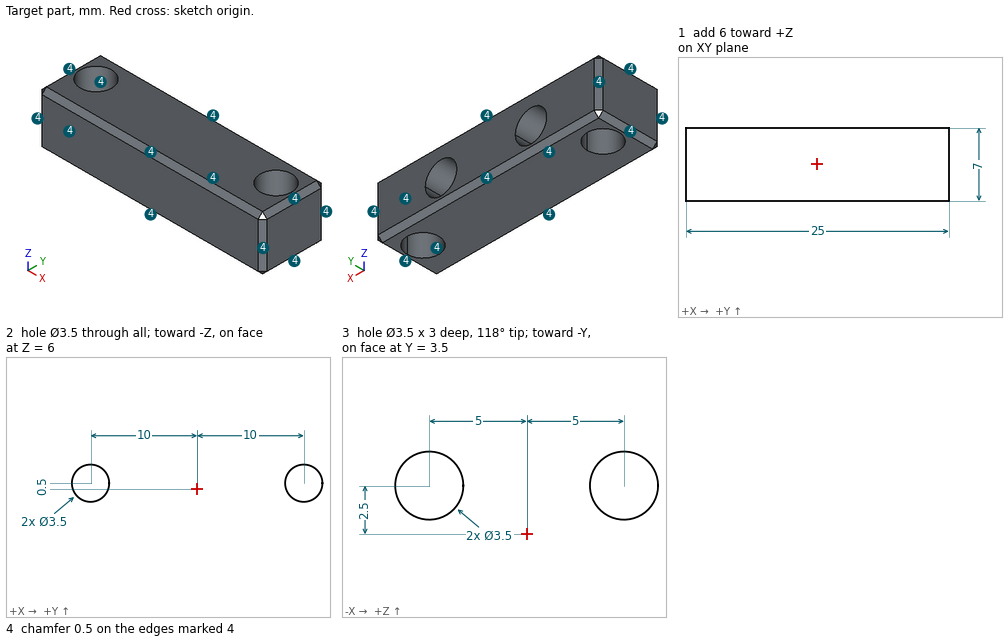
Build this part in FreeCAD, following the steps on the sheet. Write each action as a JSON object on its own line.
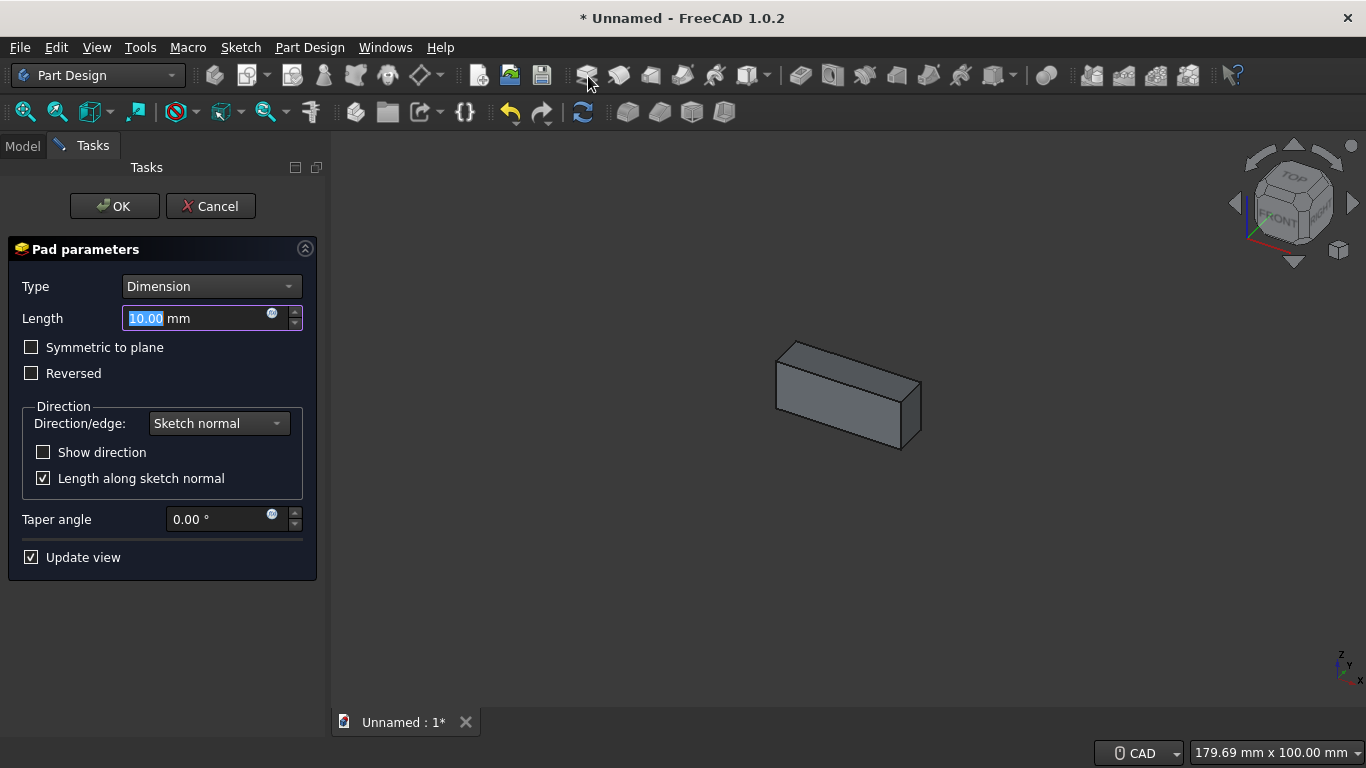
{"action": "type", "text": "6"}
{"action": "key", "text": "Tab"}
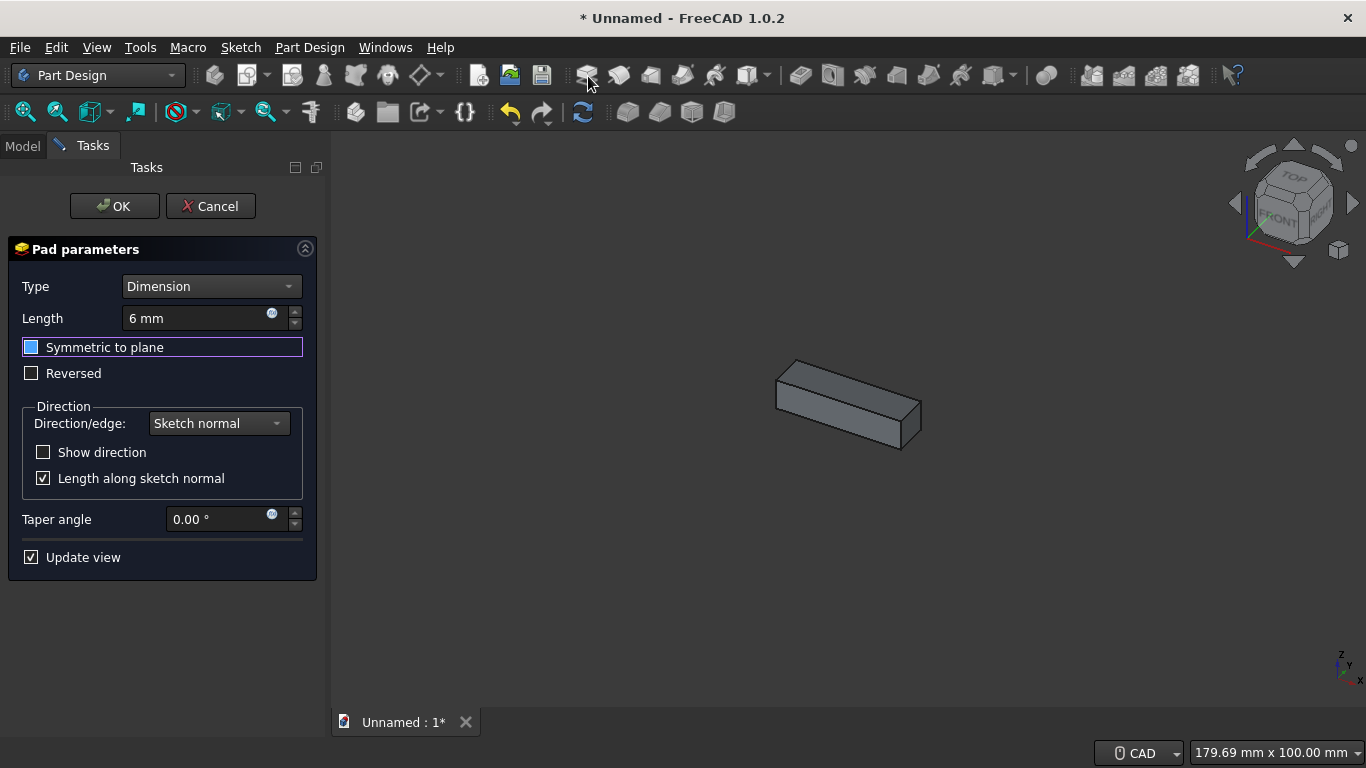
{"action": "left_click", "coordinate": [115, 206]}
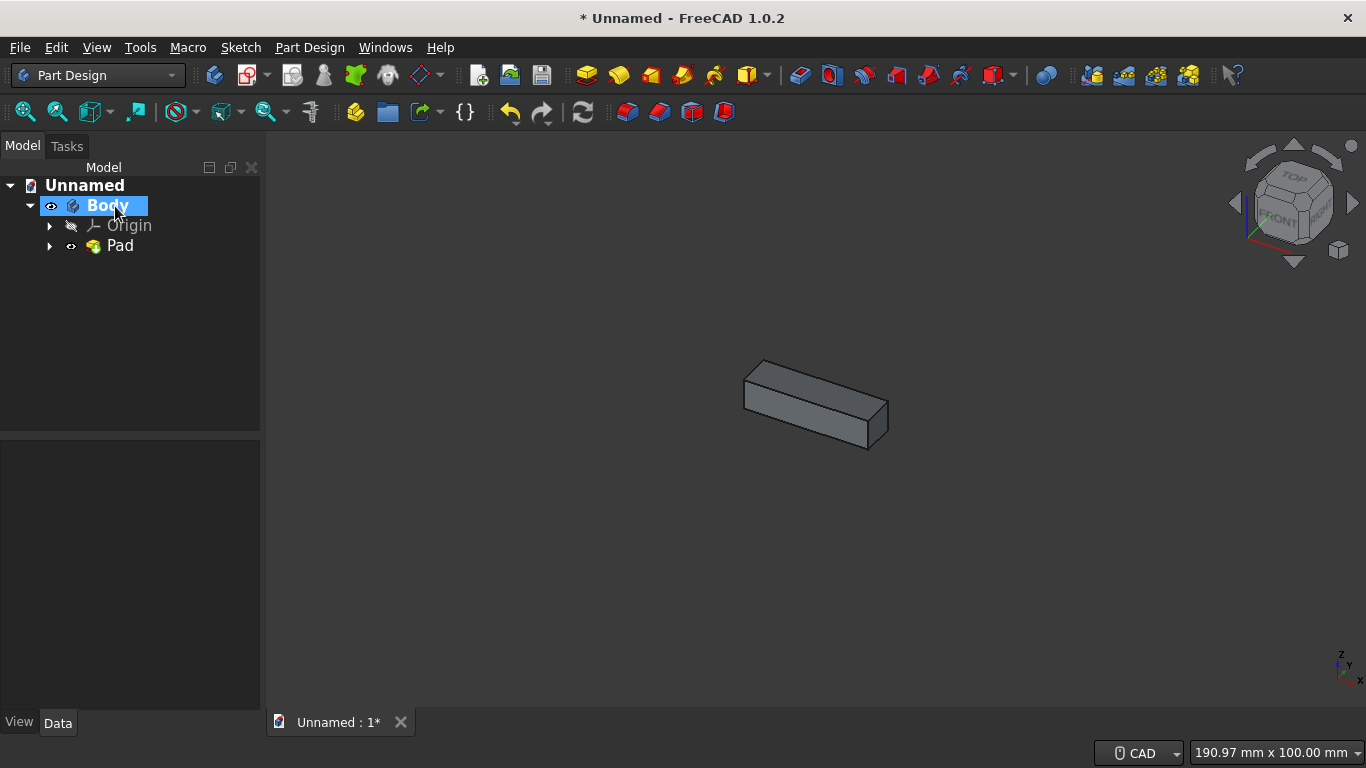
{"action": "left_click", "coordinate": [26, 112]}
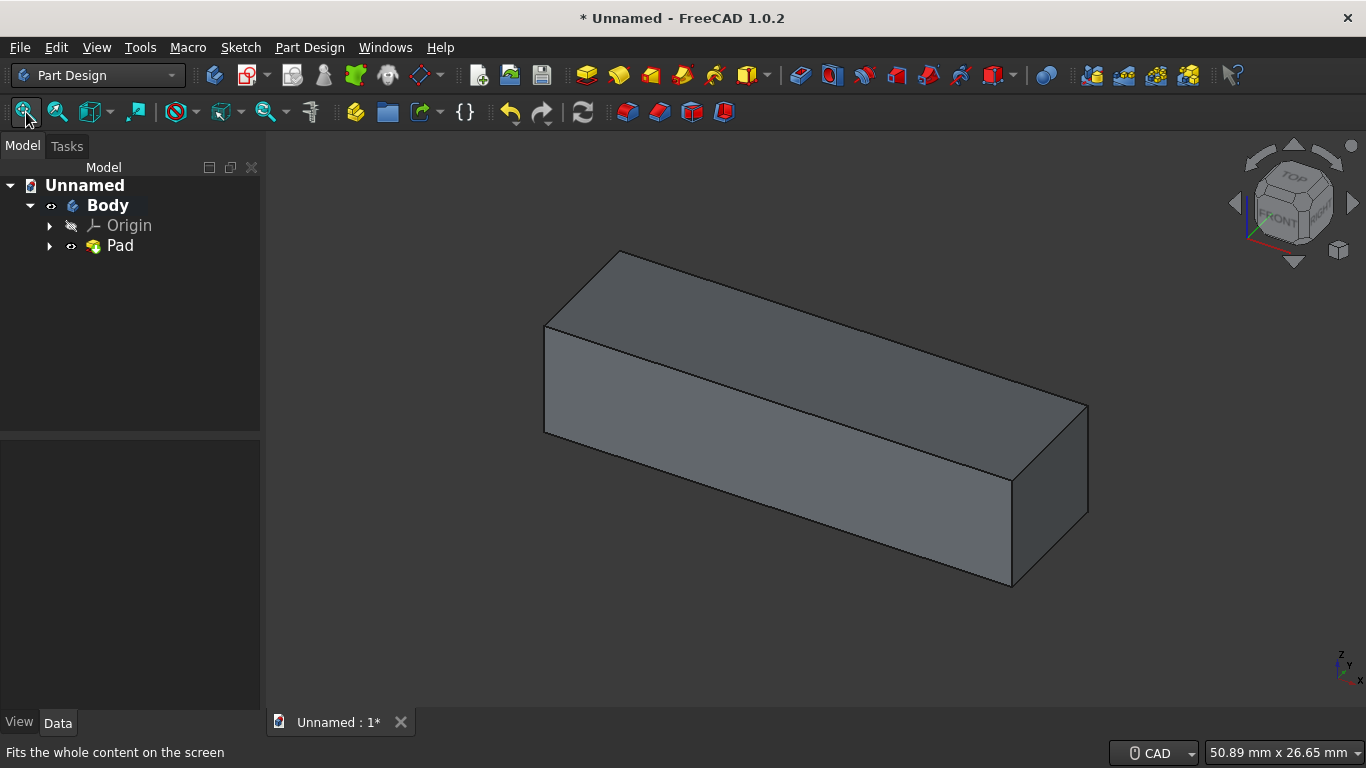
{"action": "left_click", "coordinate": [950, 409]}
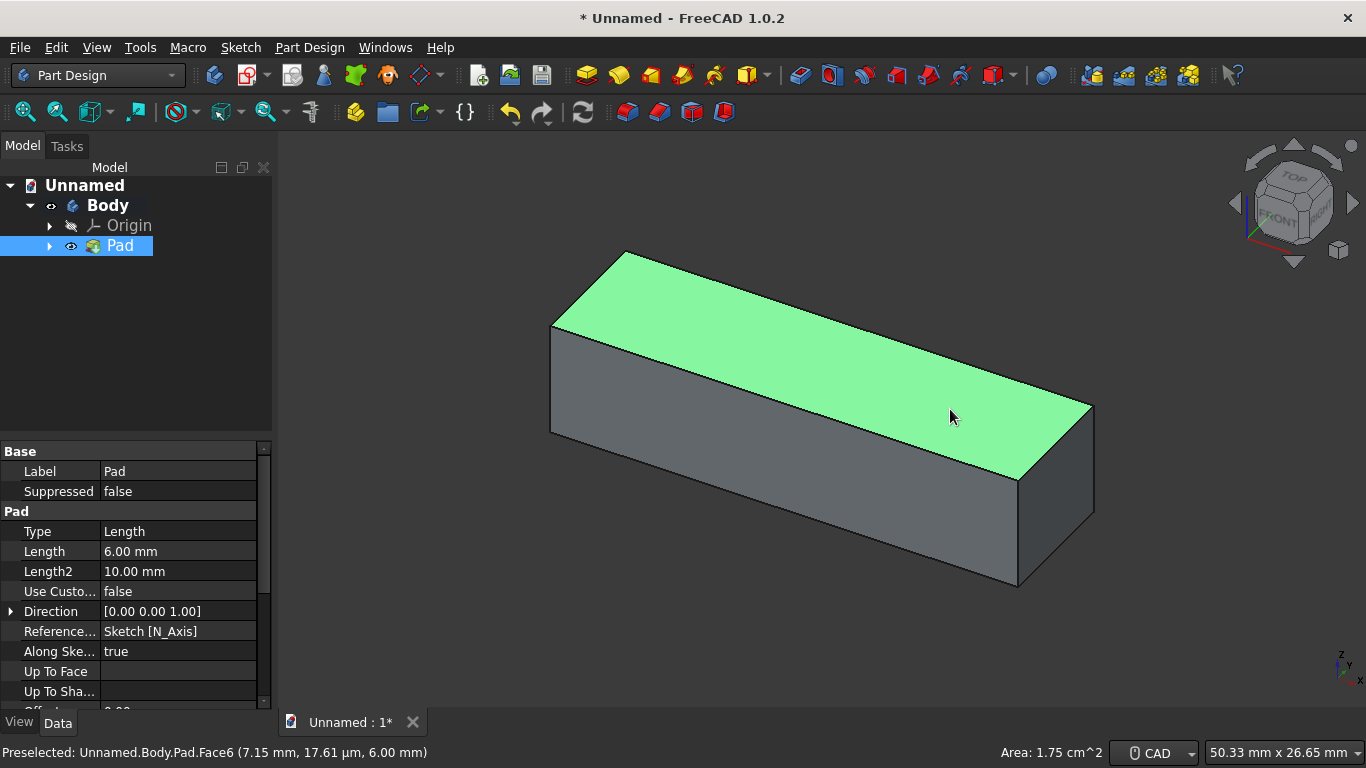
{"action": "left_click", "coordinate": [248, 76]}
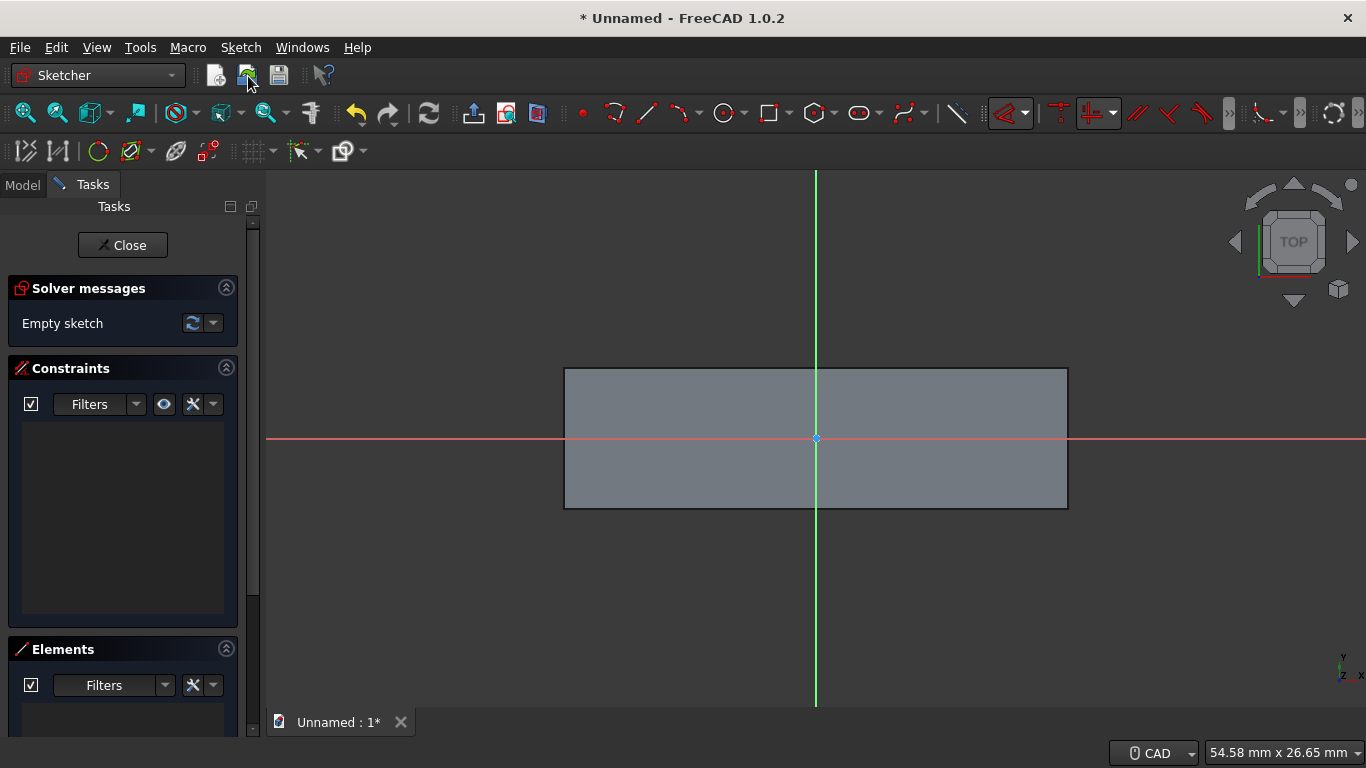
{"action": "scroll", "coordinate": [955, 408], "scroll_direction": "up", "scroll_amount": 2}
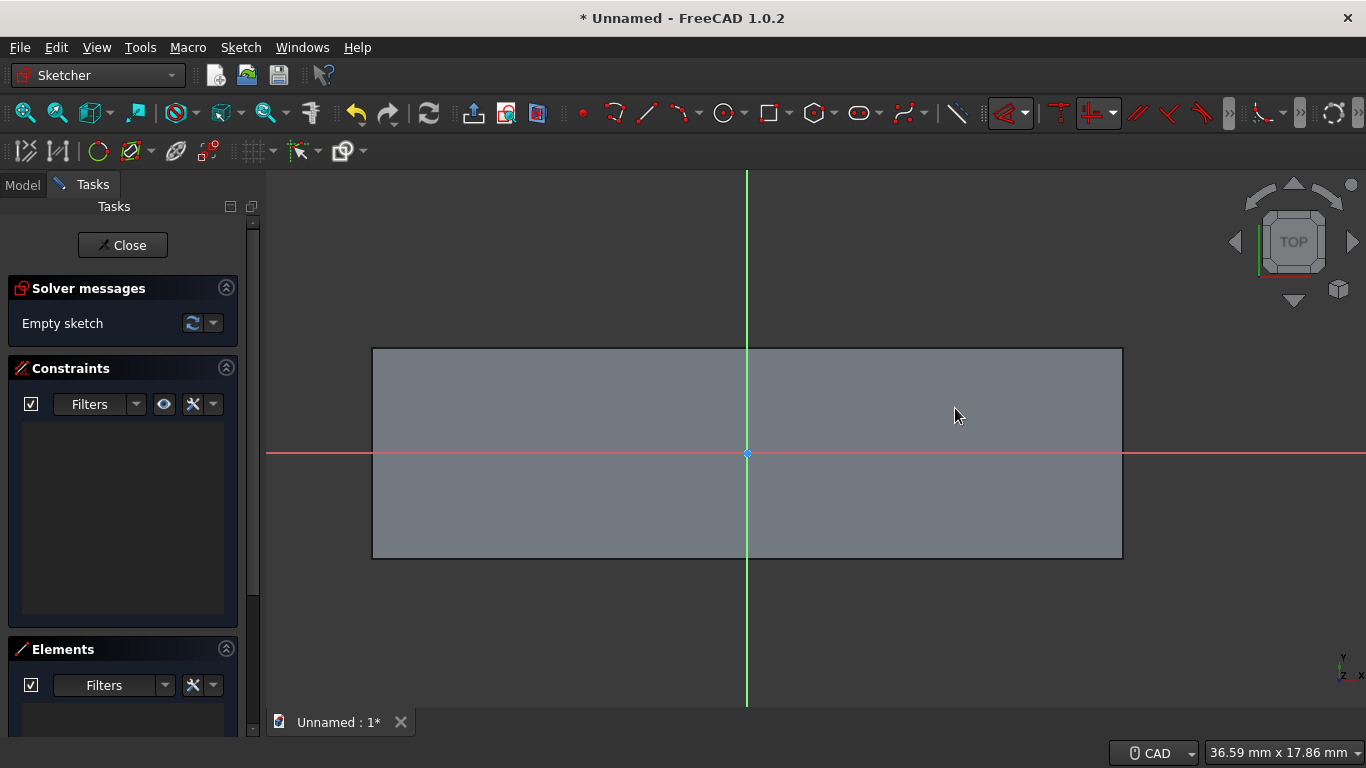
{"action": "left_click", "coordinate": [724, 114]}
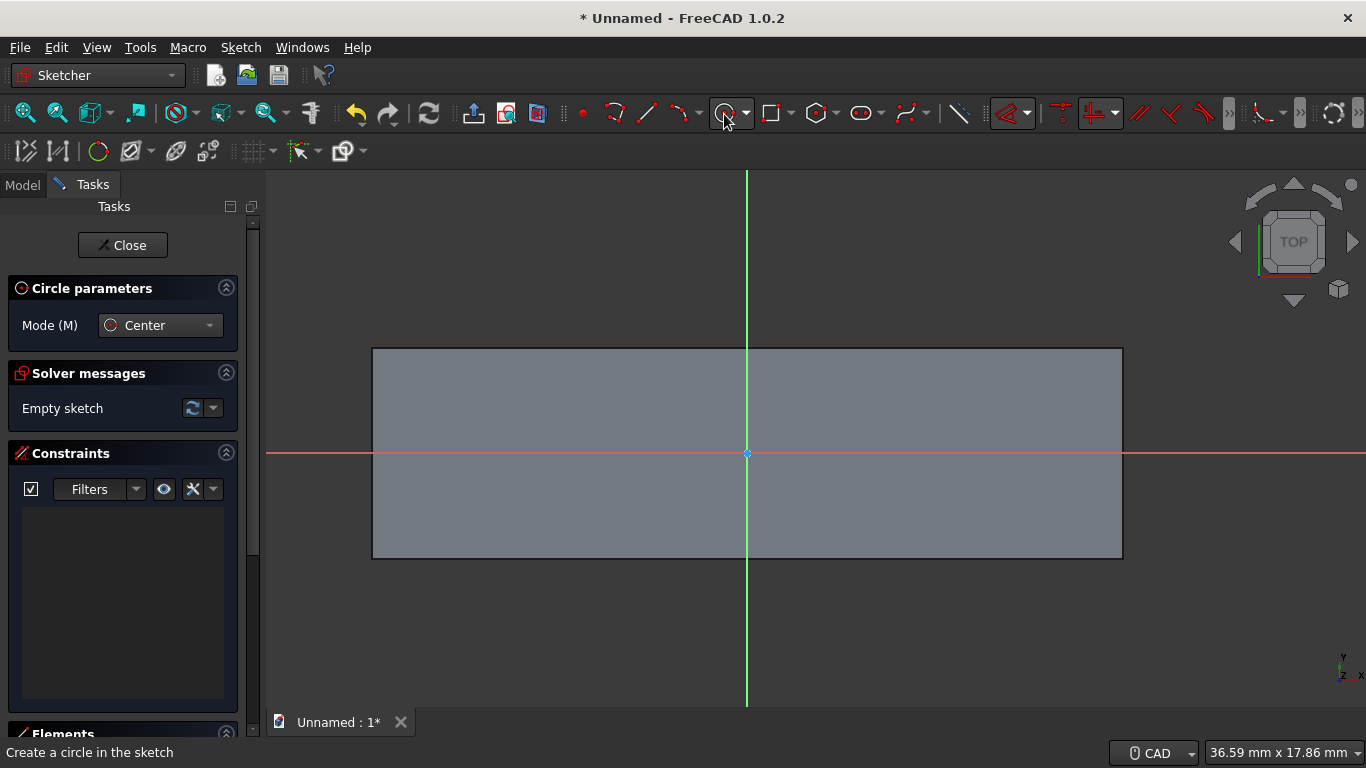
{"action": "left_click", "coordinate": [447, 438]}
{"action": "mouse_move", "coordinate": [484, 401]}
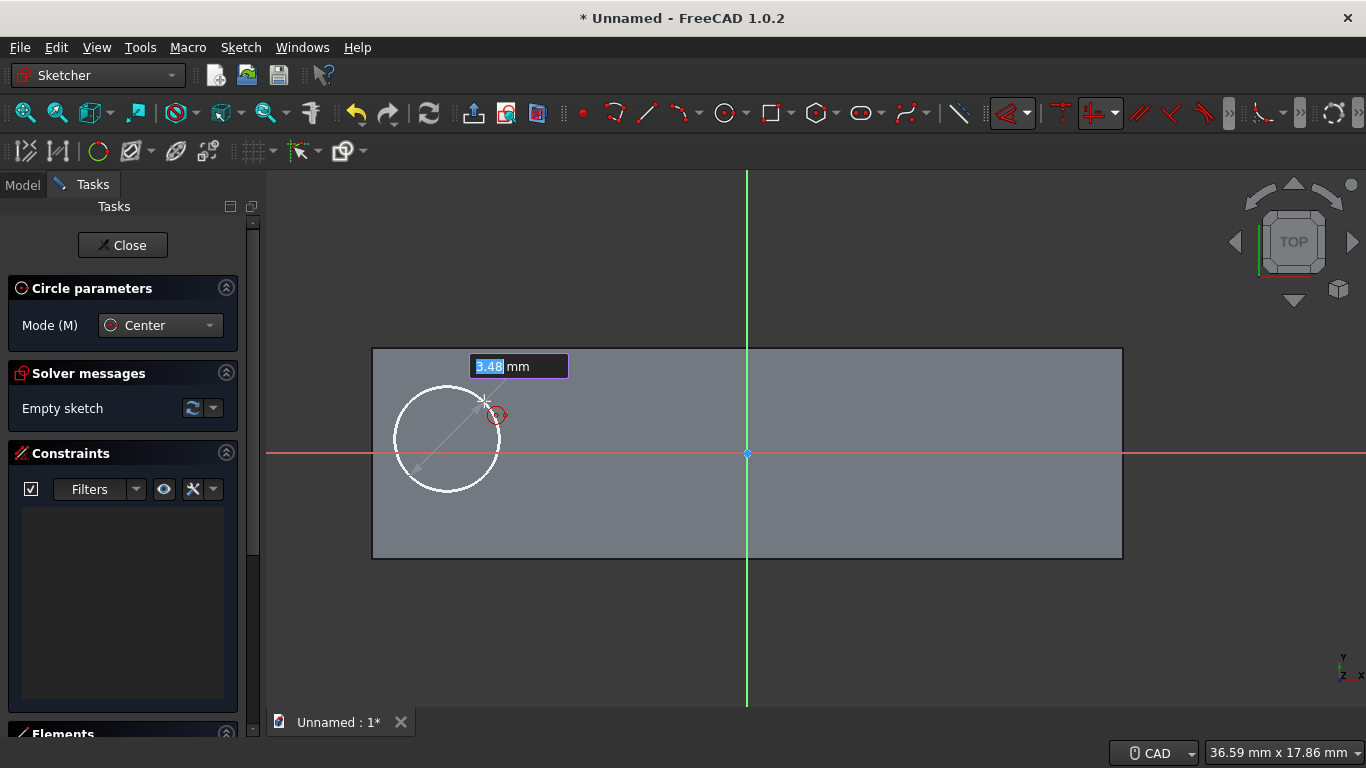
{"action": "type", "text": "3.5"}
{"action": "key", "text": "Return"}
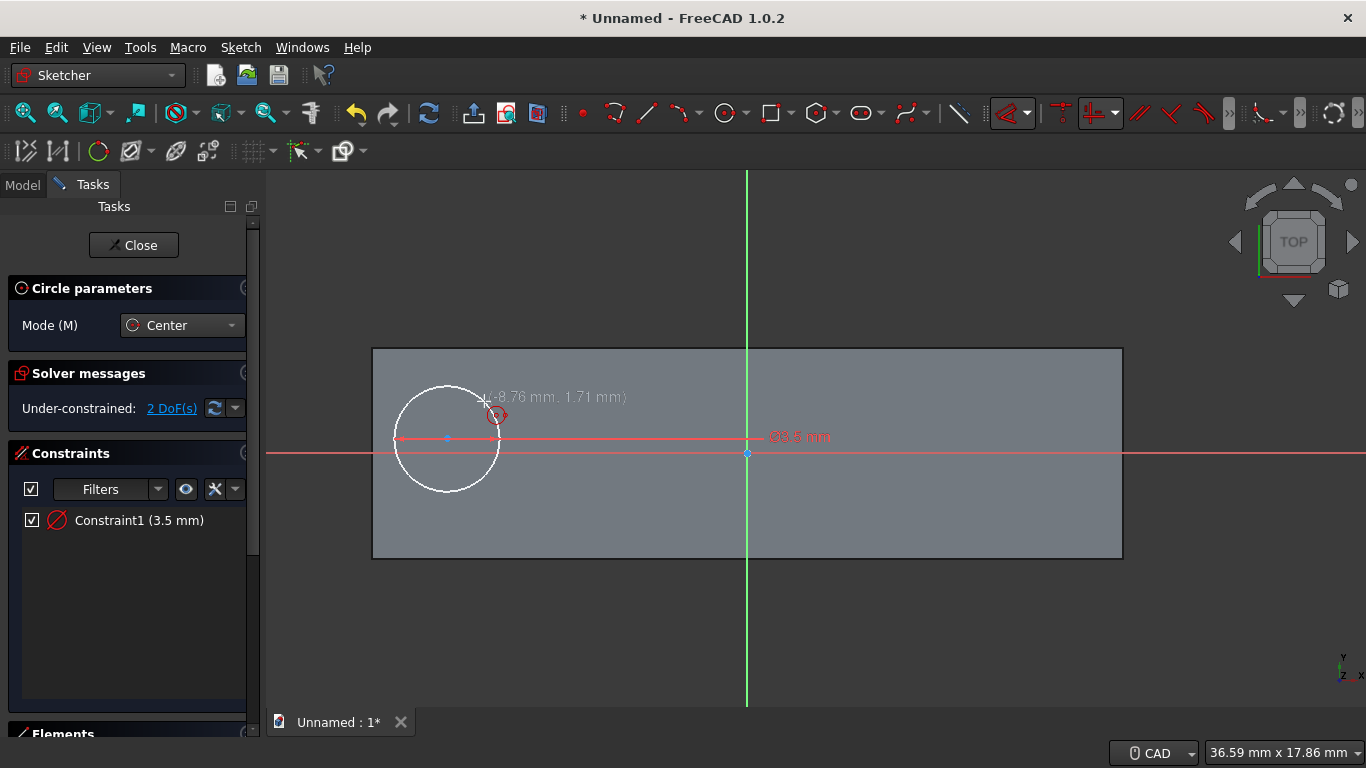
{"action": "left_click", "coordinate": [1048, 438]}
{"action": "mouse_move", "coordinate": [1085, 401]}